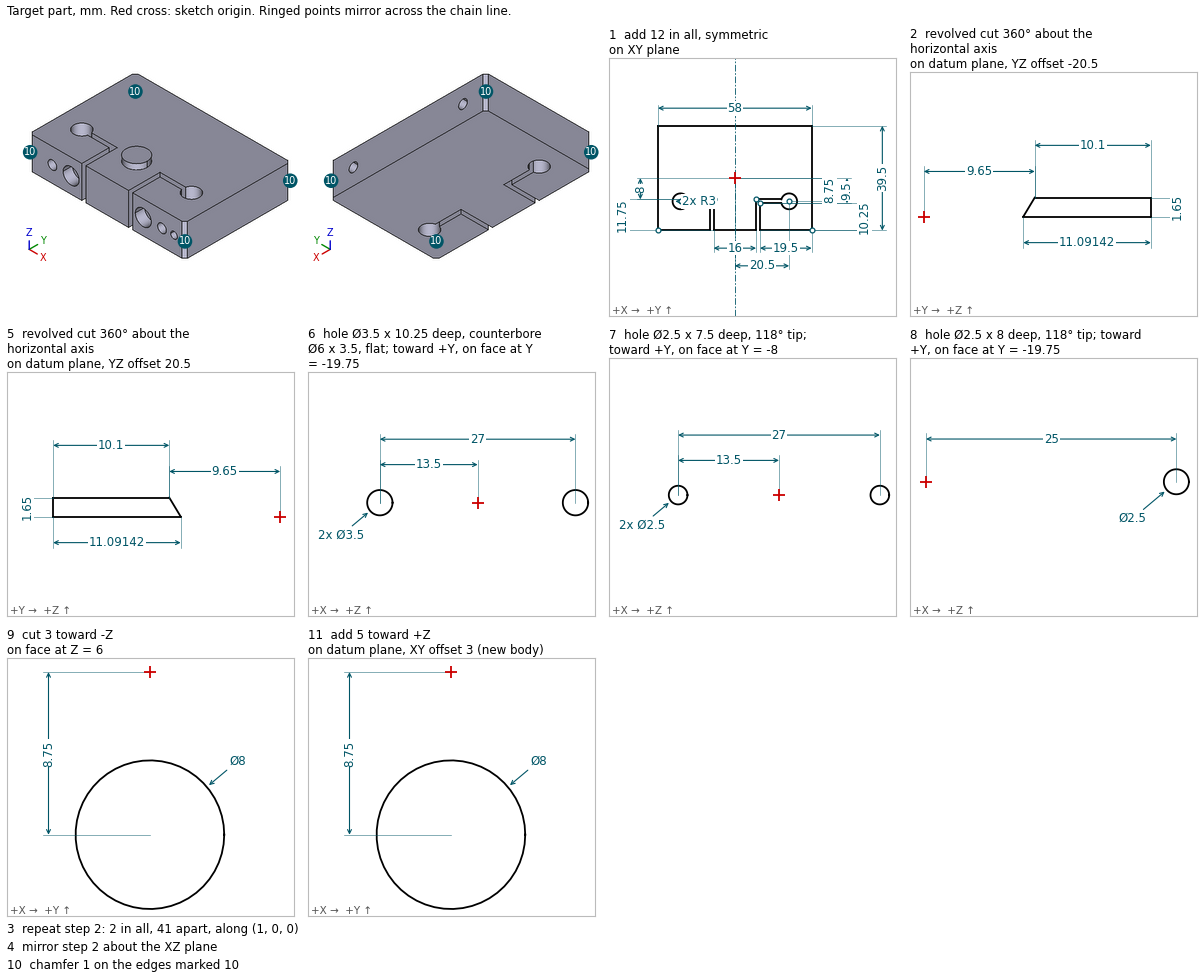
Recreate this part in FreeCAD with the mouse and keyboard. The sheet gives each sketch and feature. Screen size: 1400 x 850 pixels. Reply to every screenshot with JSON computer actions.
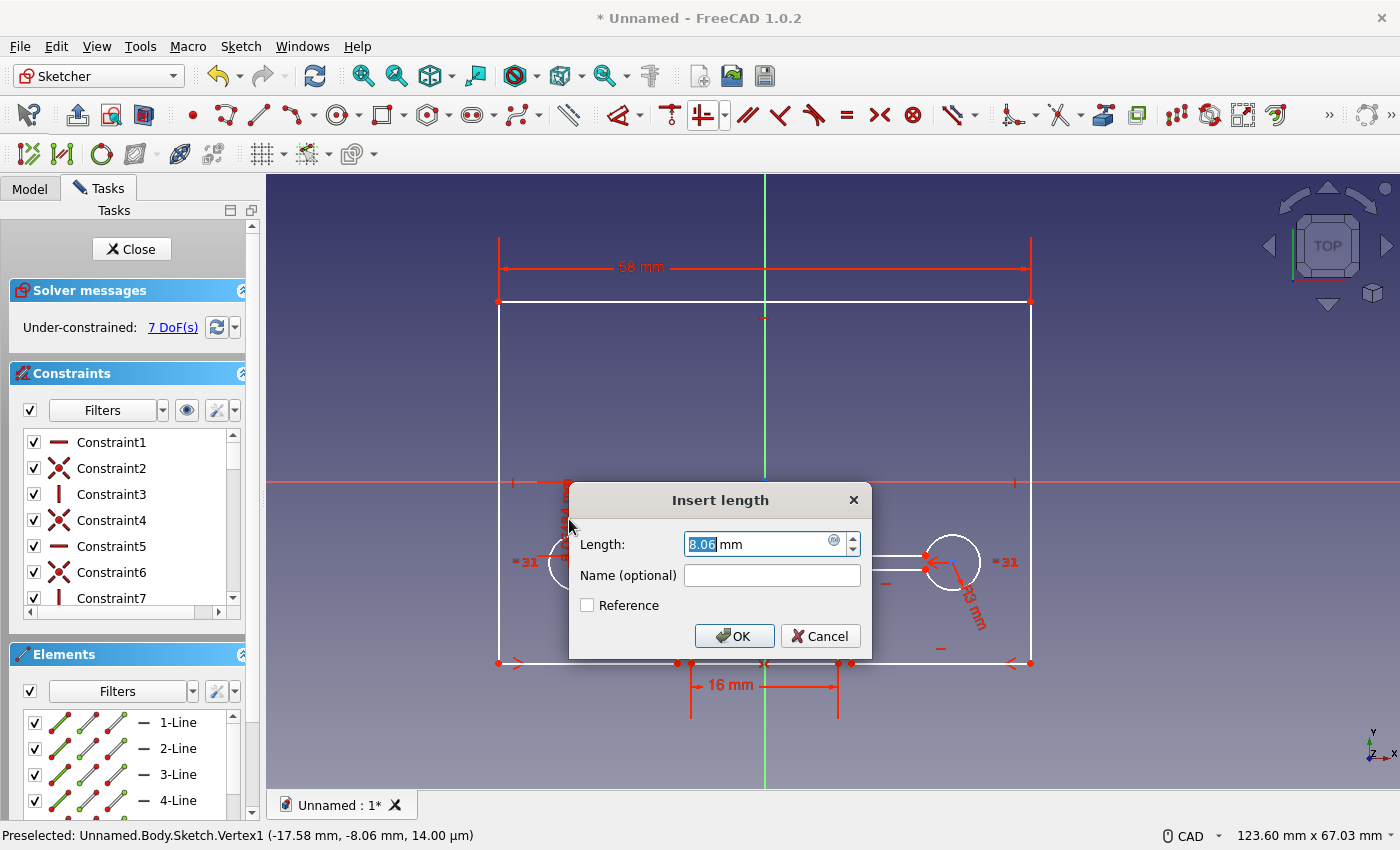
{"action": "type", "text": "8"}
{"action": "key", "text": "Return"}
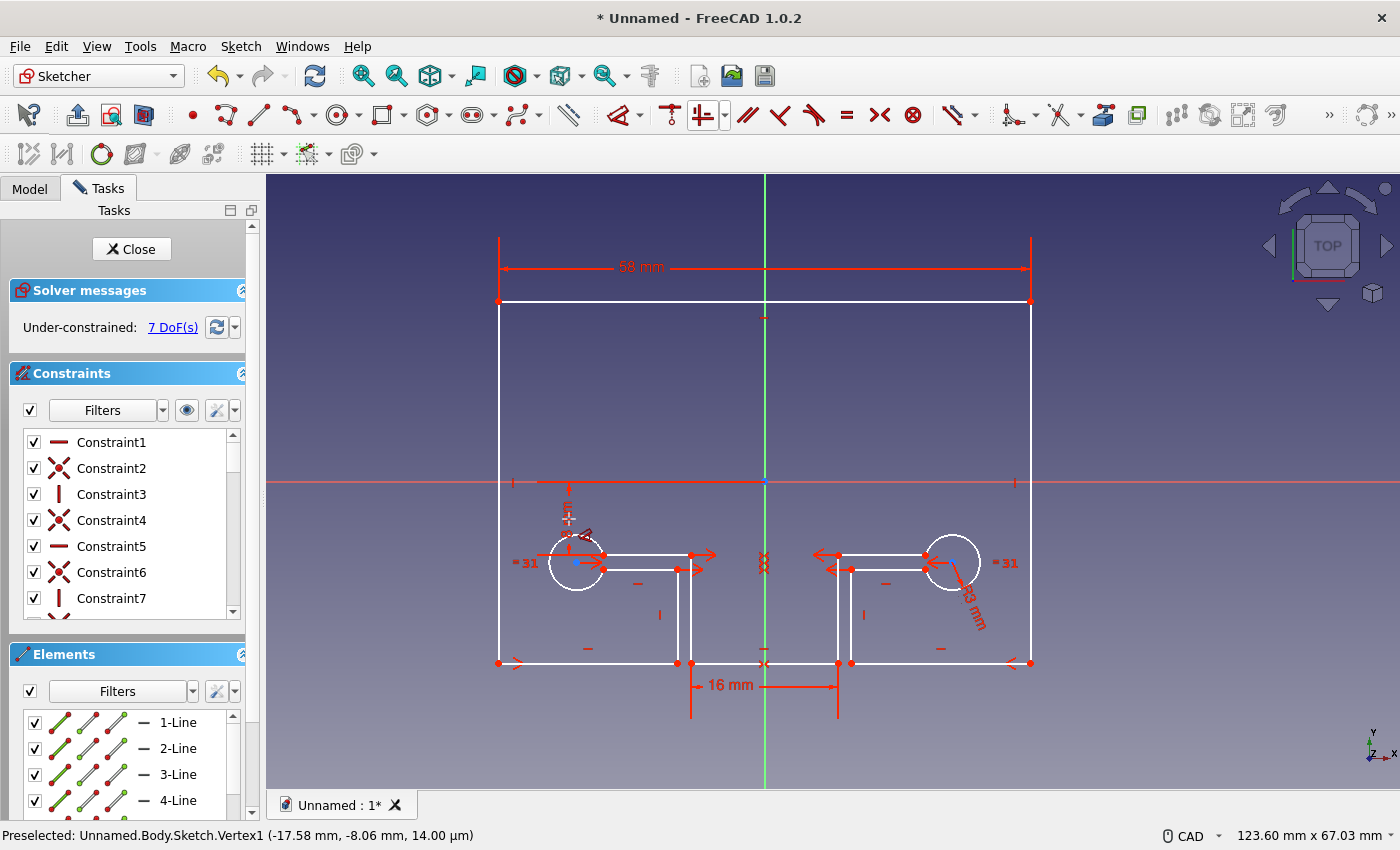
{"action": "left_click", "coordinate": [905, 664]}
{"action": "left_click", "coordinate": [941, 698]}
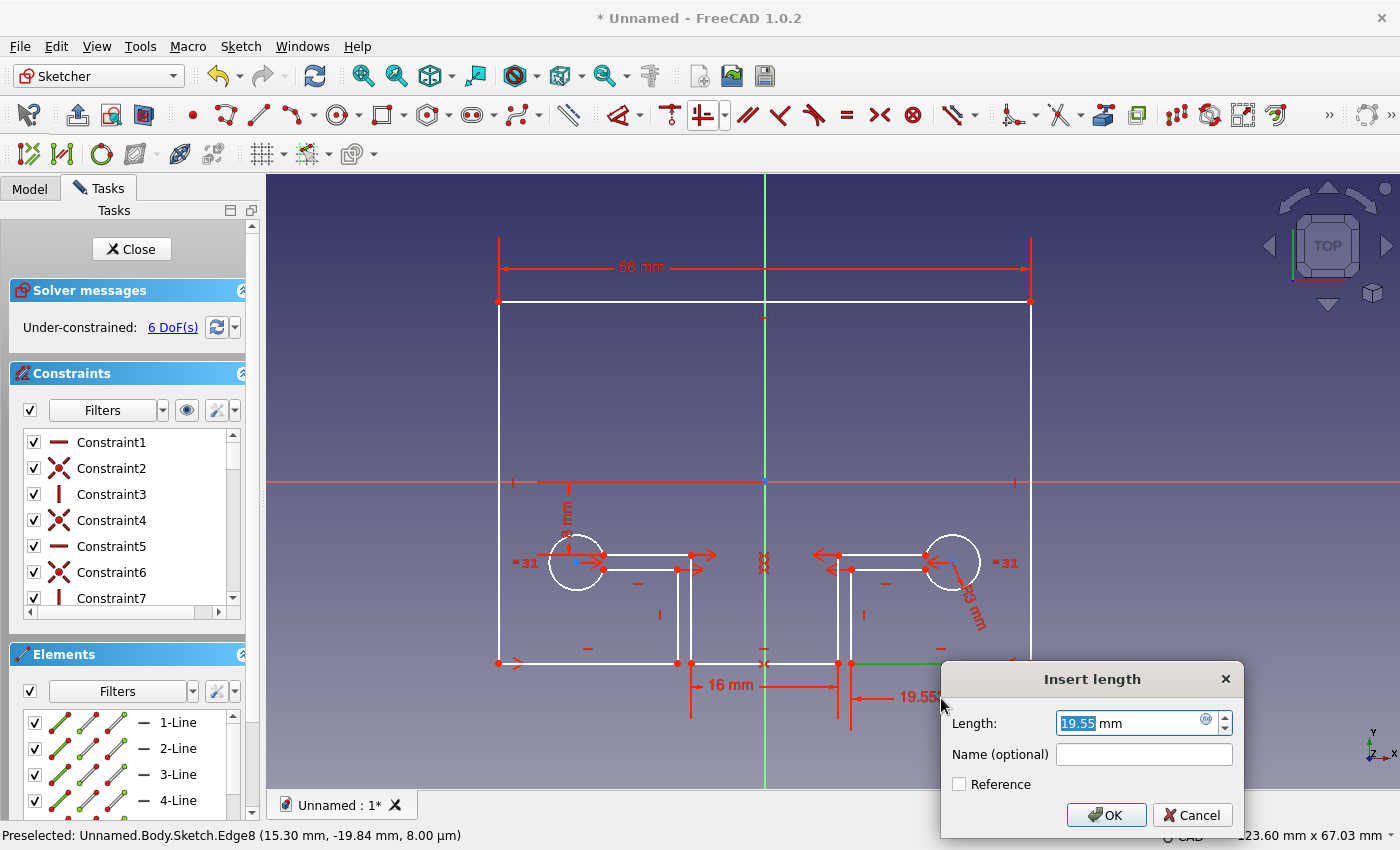
{"action": "type", "text": "19.5"}
{"action": "key", "text": "Return"}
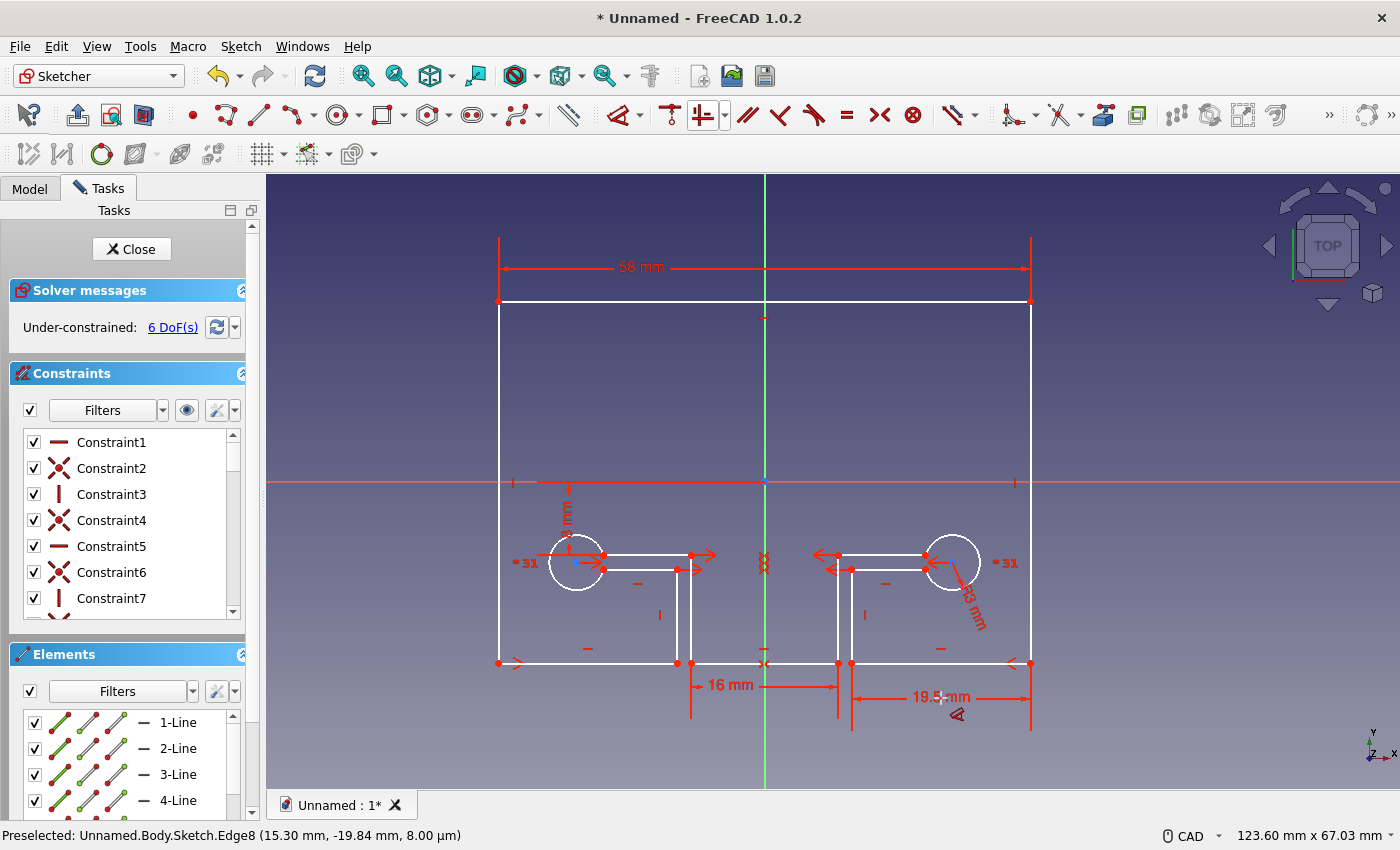
{"action": "left_click", "coordinate": [1031, 555]}
{"action": "left_click", "coordinate": [1065, 399]}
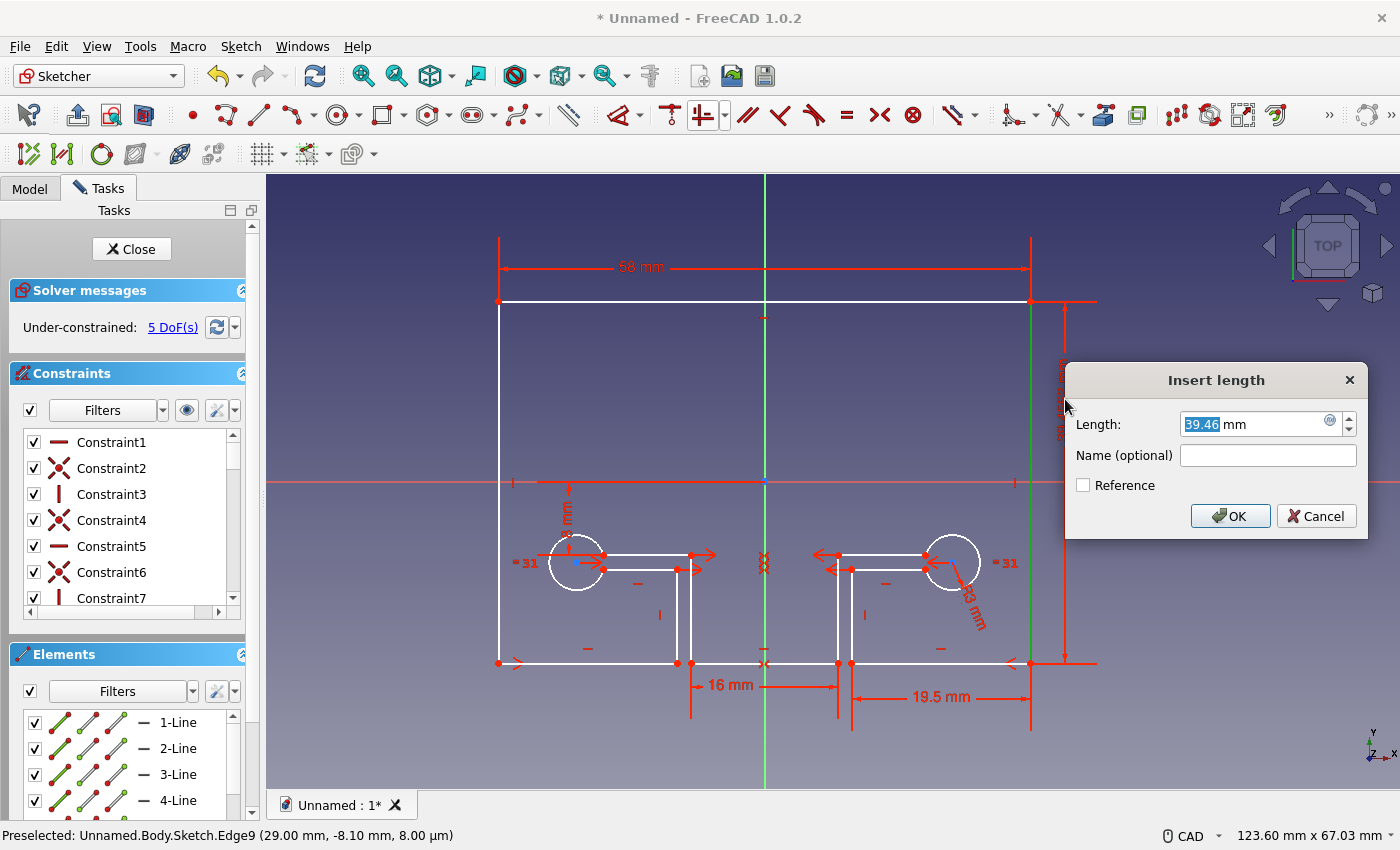
{"action": "type", "text": "39.5"}
{"action": "key", "text": "Return"}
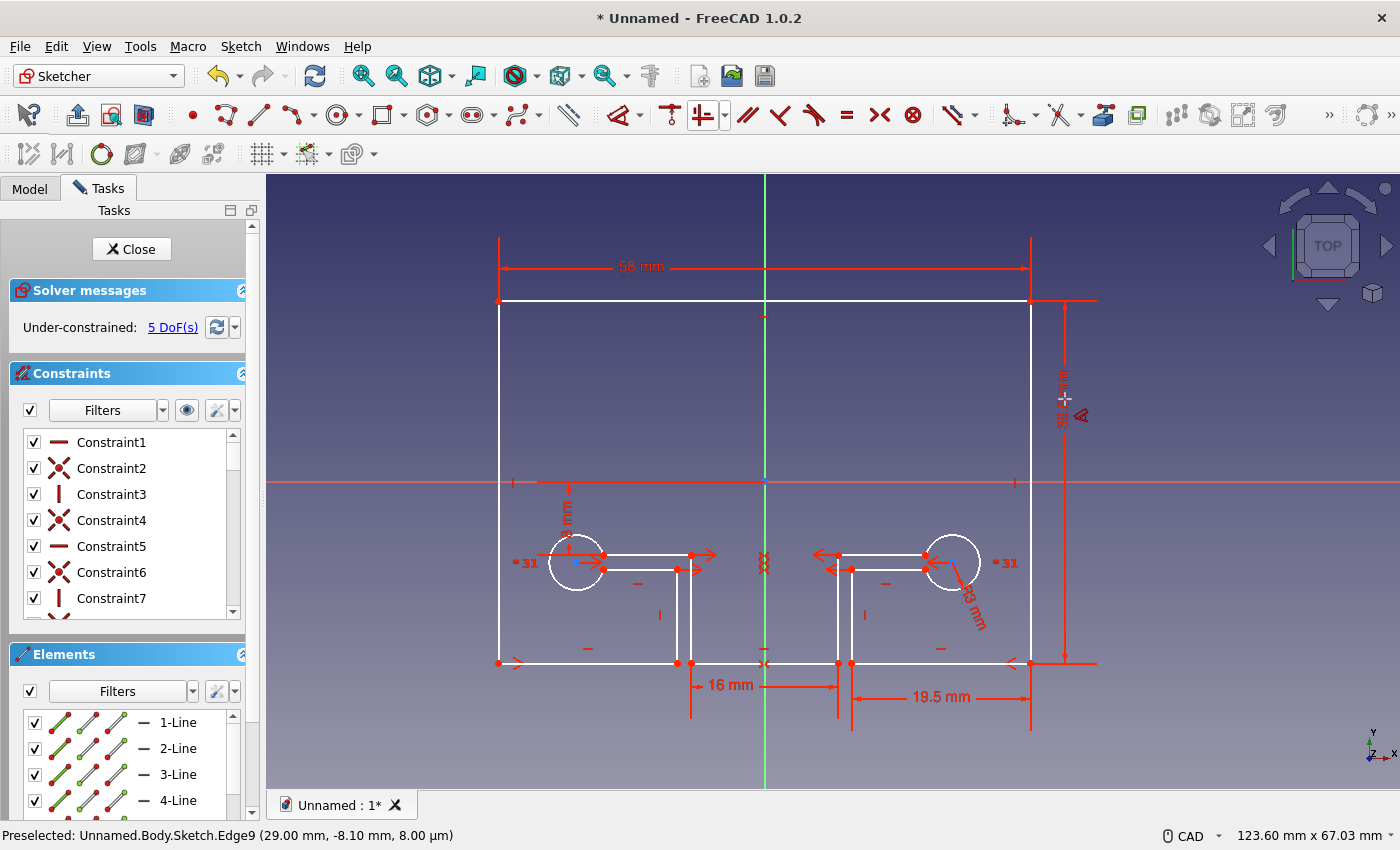
{"action": "left_click", "coordinate": [926, 570]}
{"action": "left_click", "coordinate": [960, 505]}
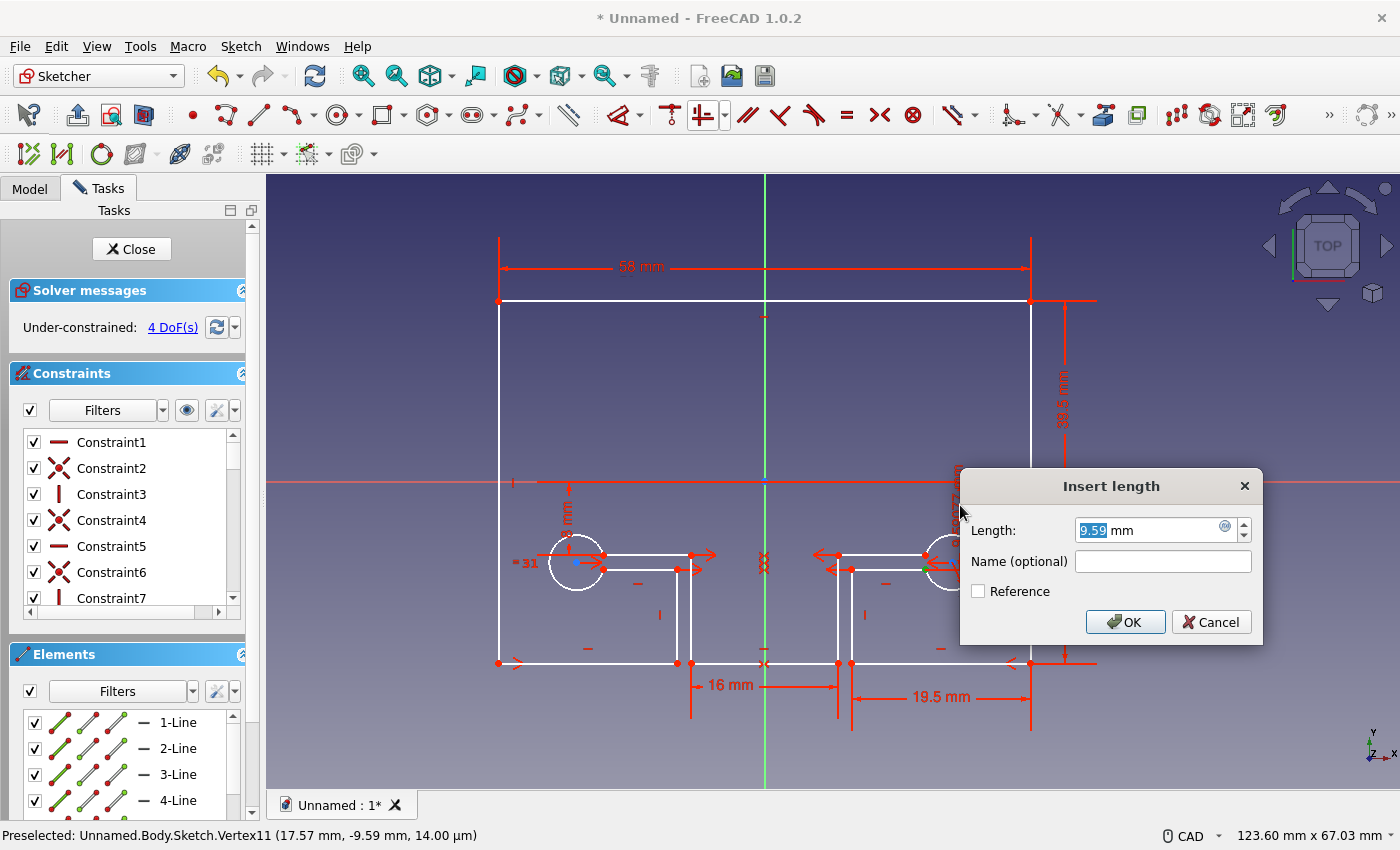
{"action": "type", "text": "9.5"}
{"action": "key", "text": "Return"}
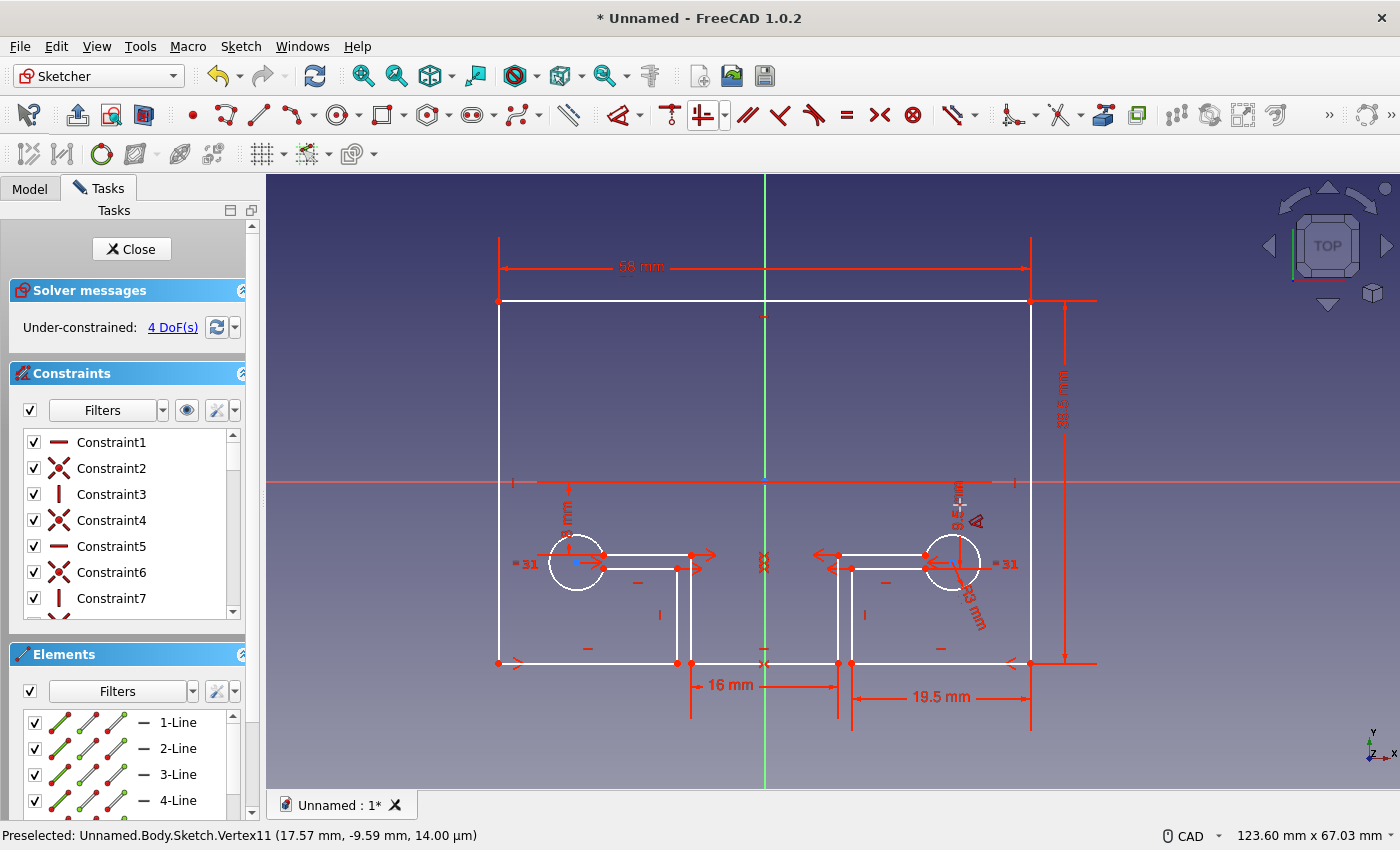
{"action": "left_click", "coordinate": [691, 588]}
{"action": "left_click", "coordinate": [657, 609]}